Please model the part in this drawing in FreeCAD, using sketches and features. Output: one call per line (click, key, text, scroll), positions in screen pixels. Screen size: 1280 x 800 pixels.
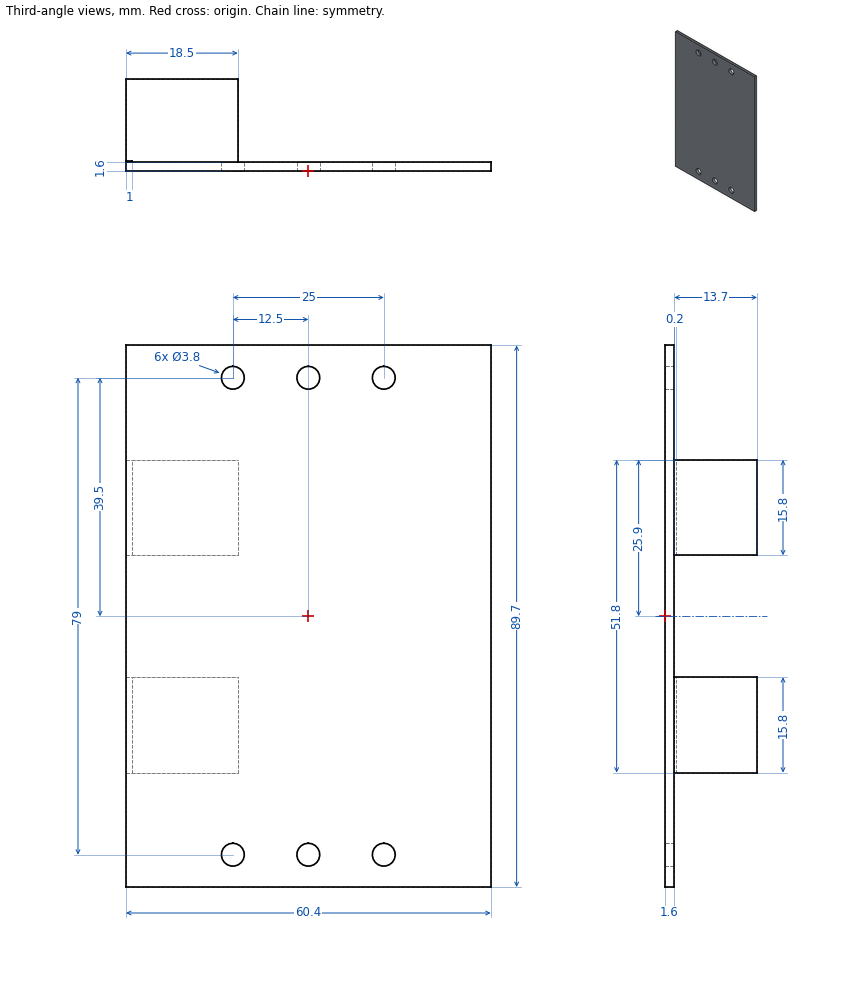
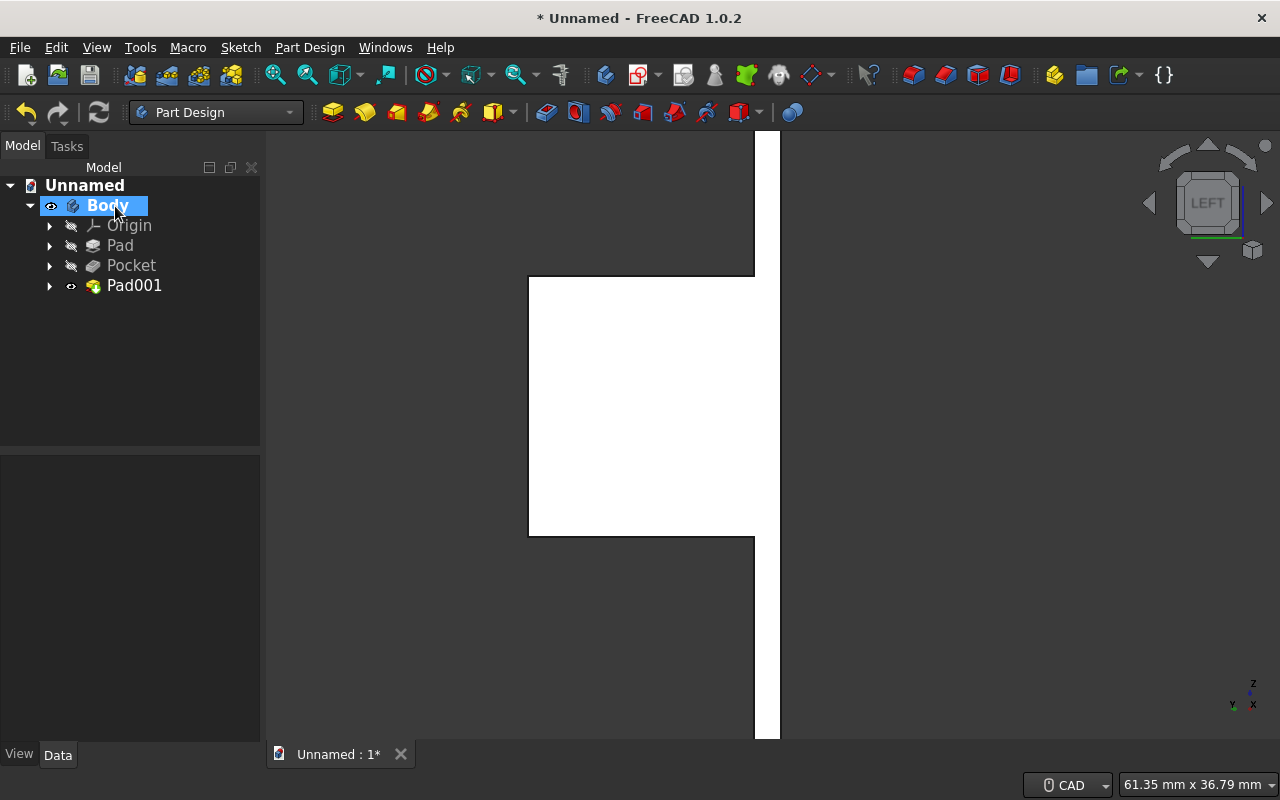
click(276, 76)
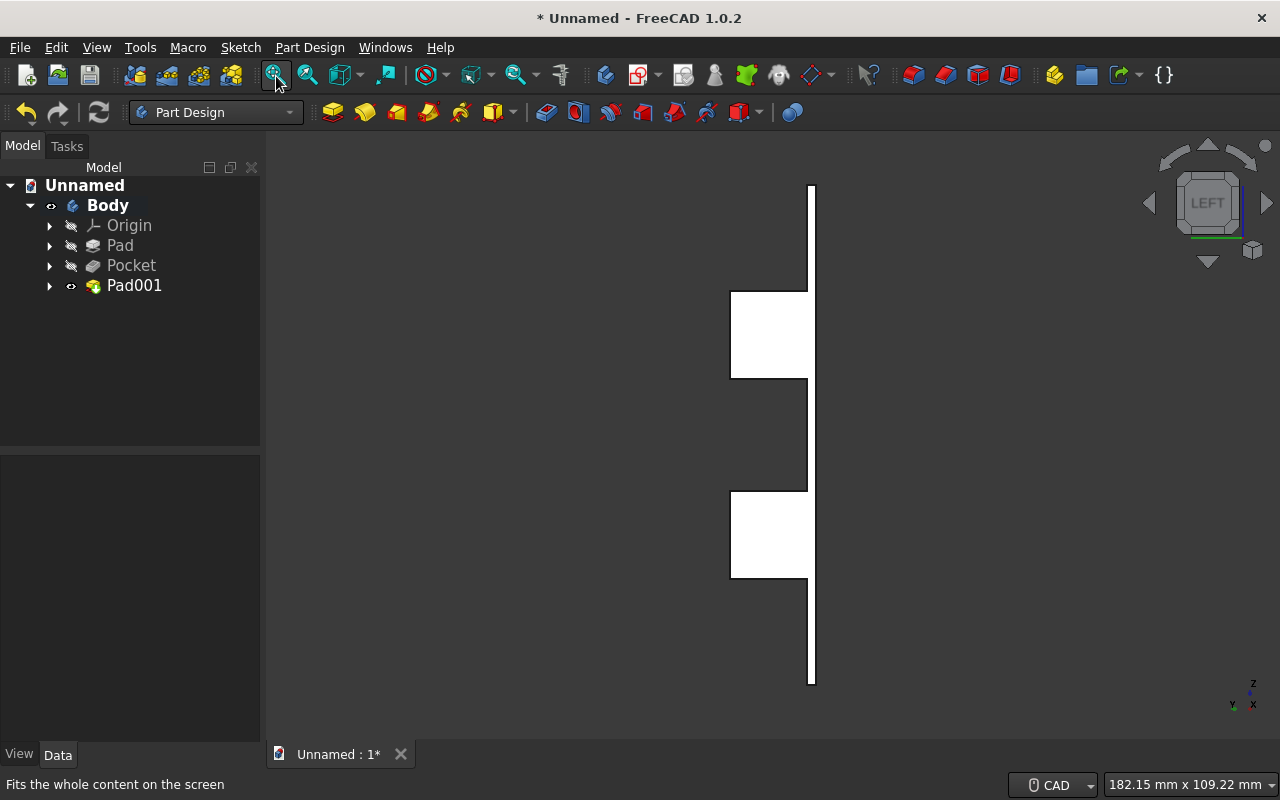
click(797, 505)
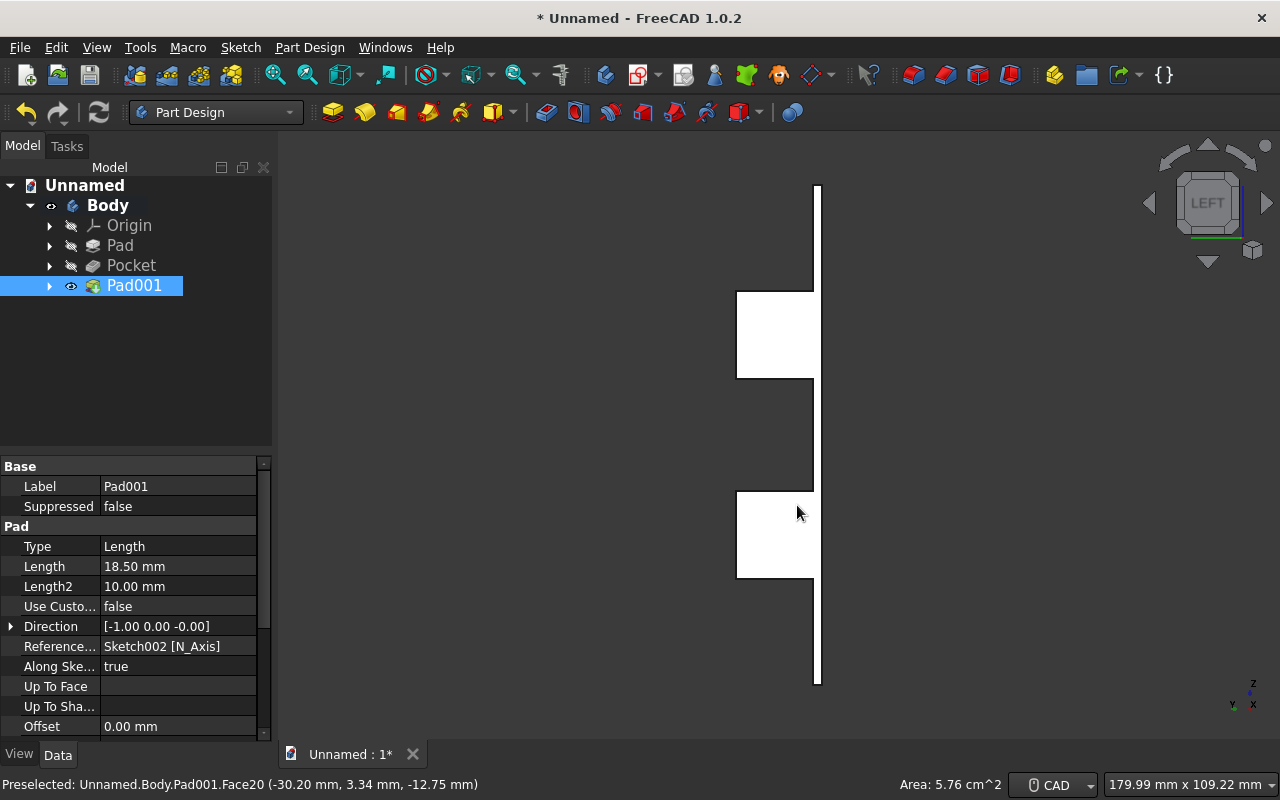
click(638, 76)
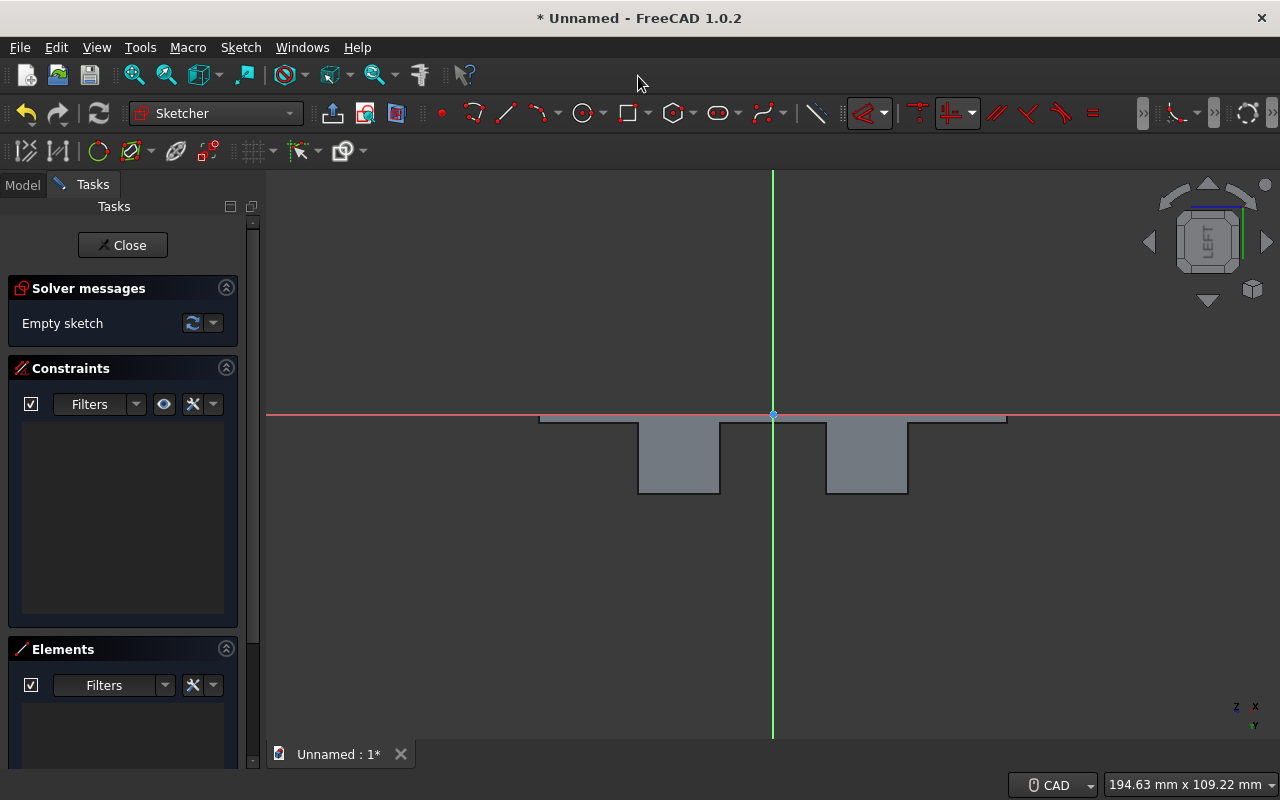
scroll(829, 391, up, 4)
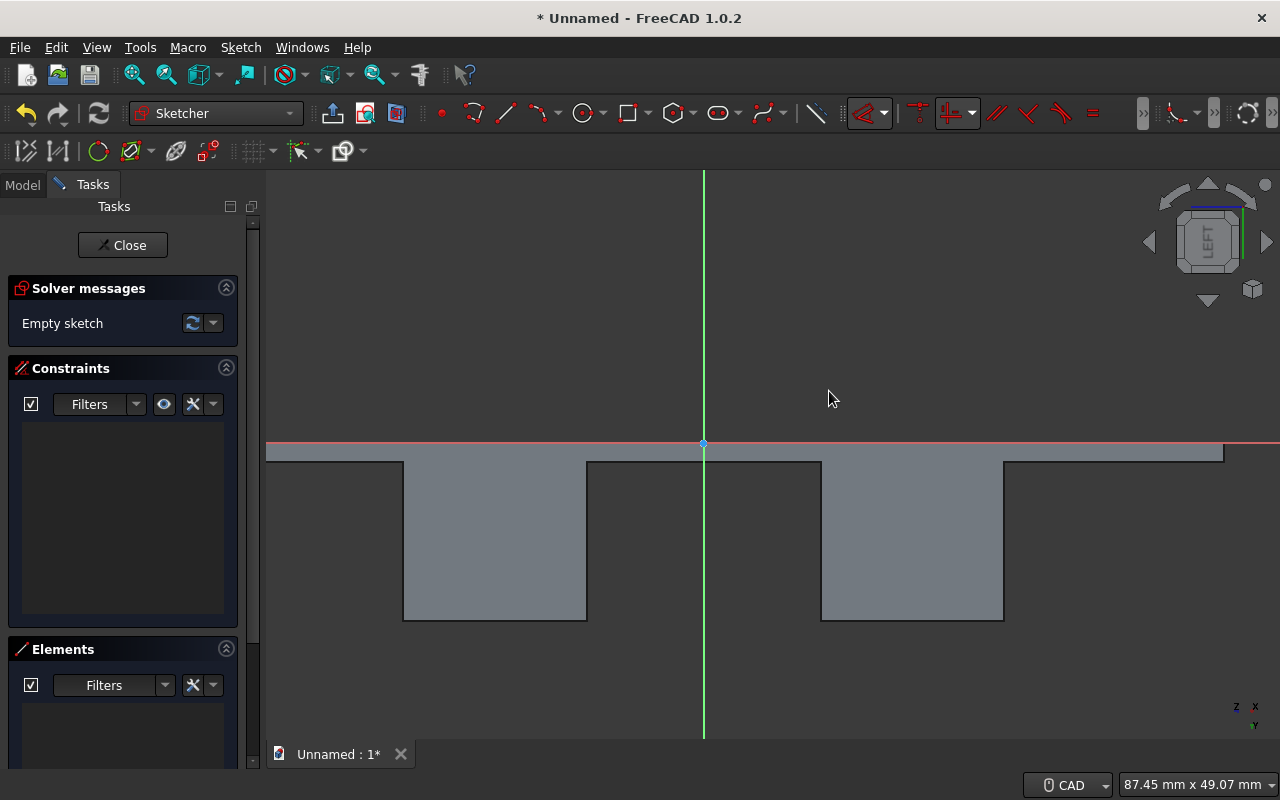
key(g)
key(r)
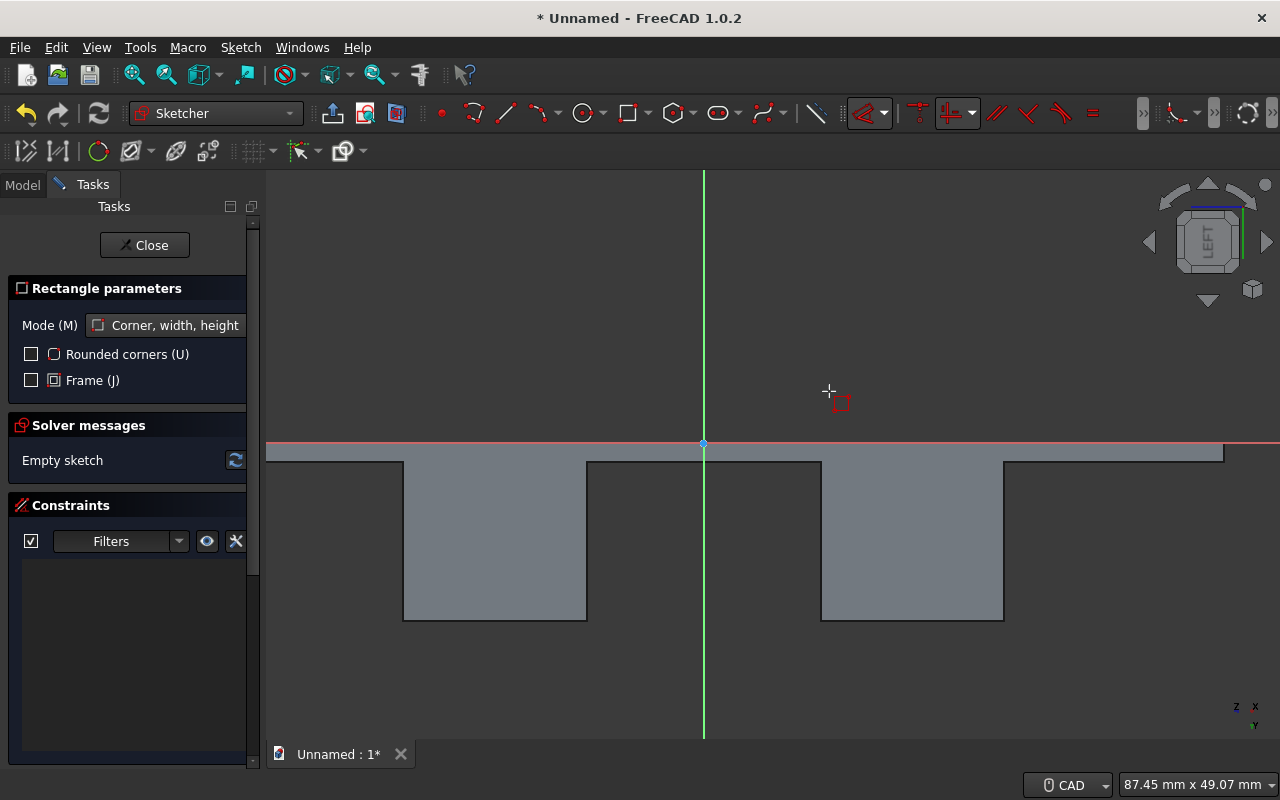
scroll(403, 462, up, 10)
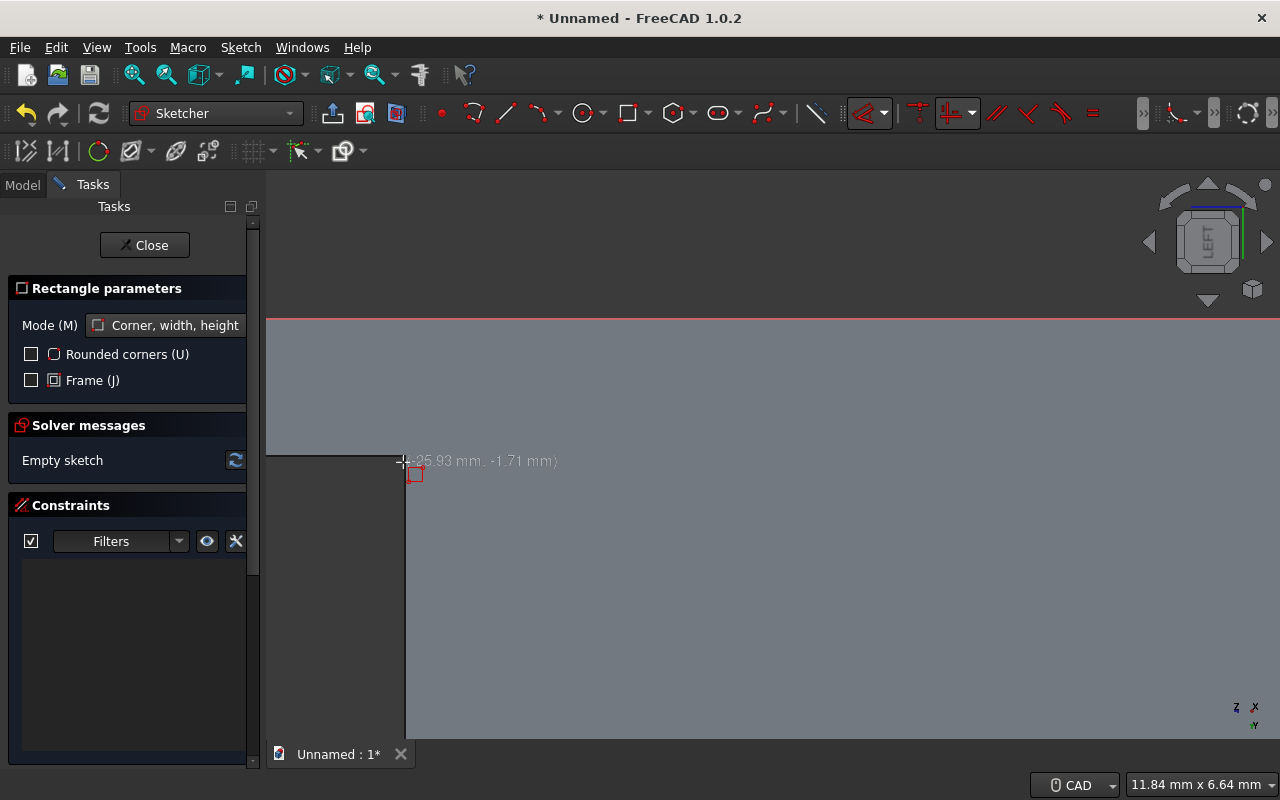
scroll(404, 464, down, 10)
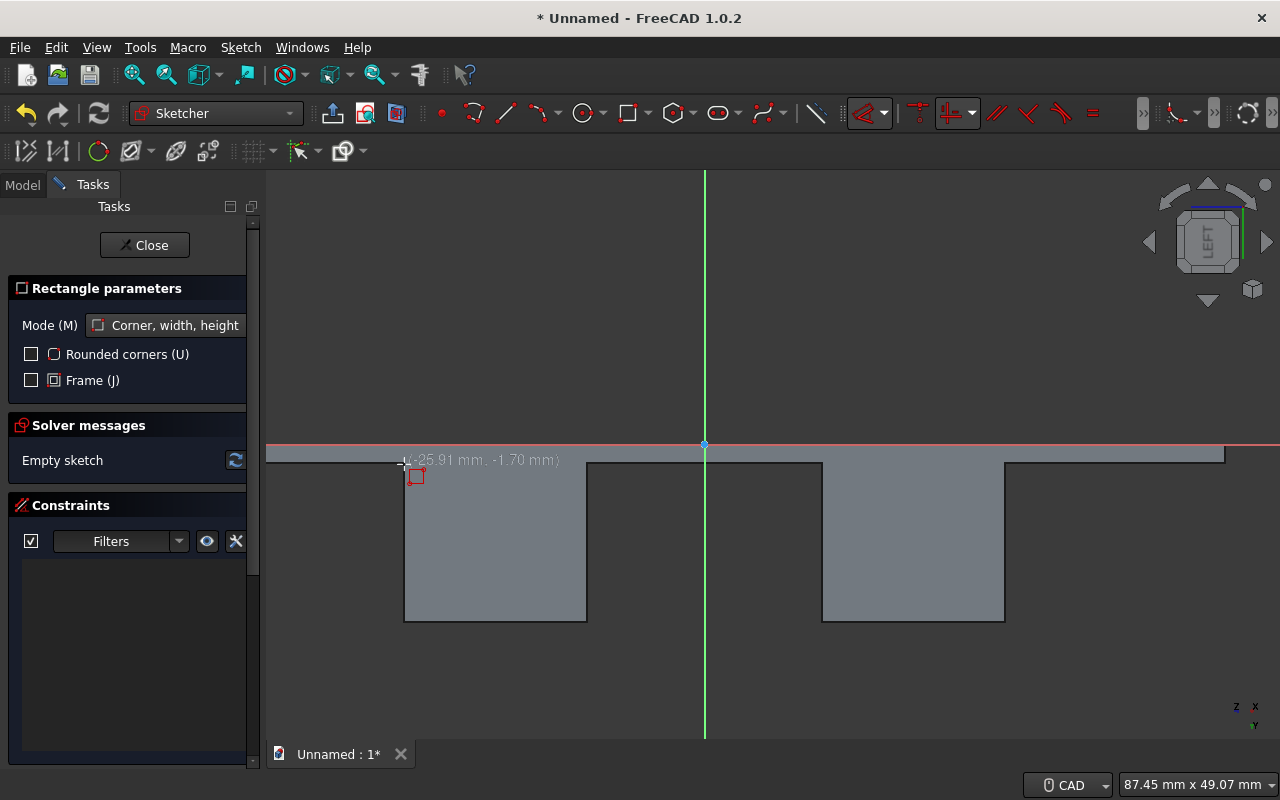
click(404, 463)
click(1005, 466)
key(Escape)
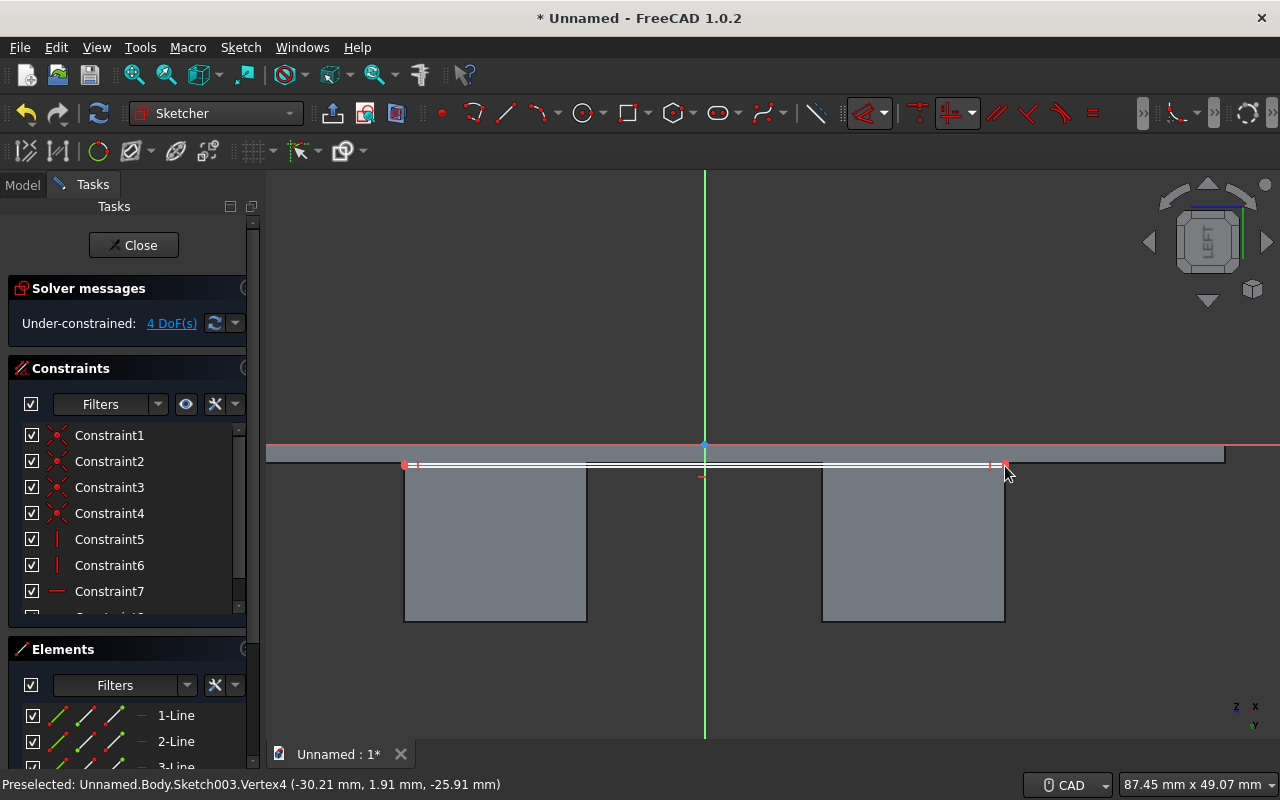
scroll(404, 465, up, 15)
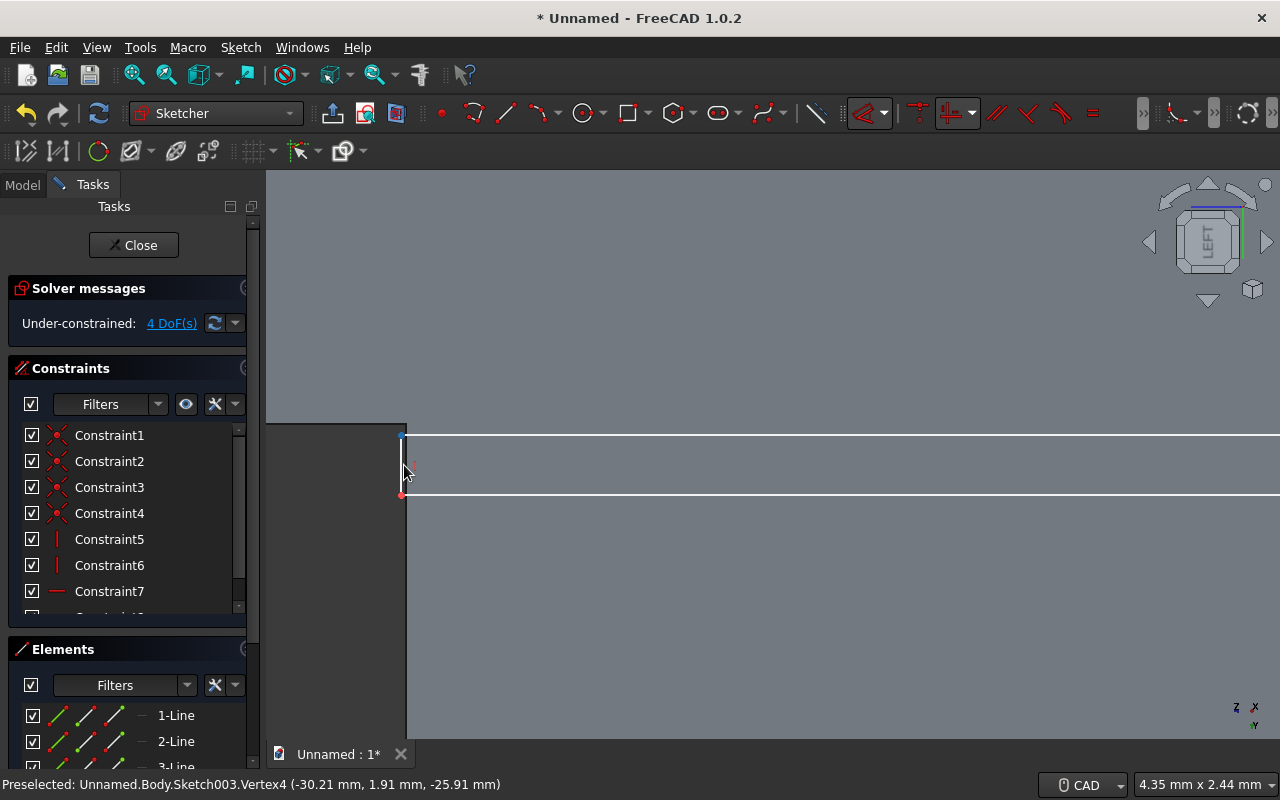
click(401, 465)